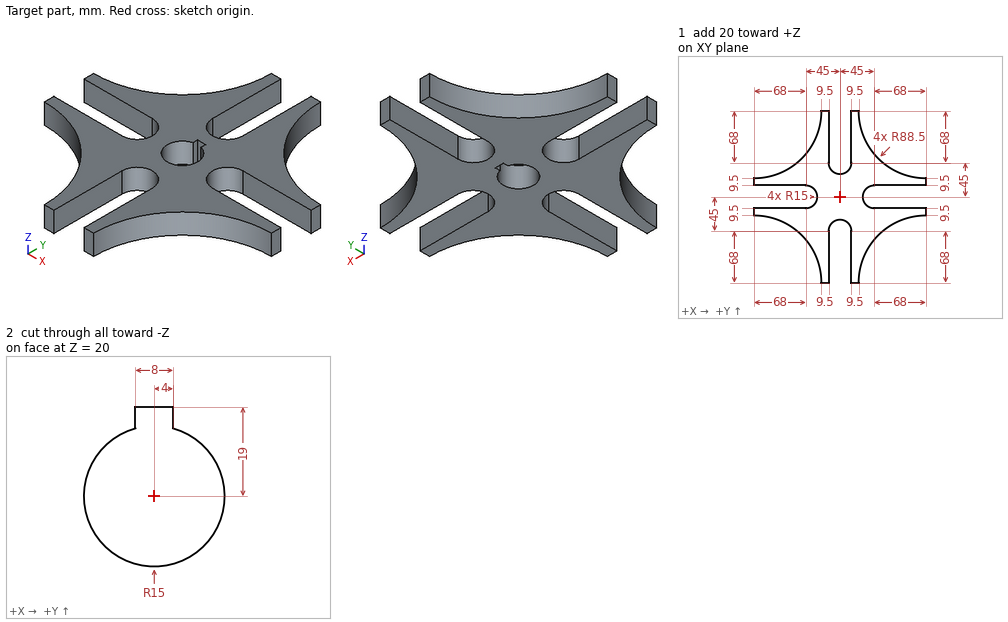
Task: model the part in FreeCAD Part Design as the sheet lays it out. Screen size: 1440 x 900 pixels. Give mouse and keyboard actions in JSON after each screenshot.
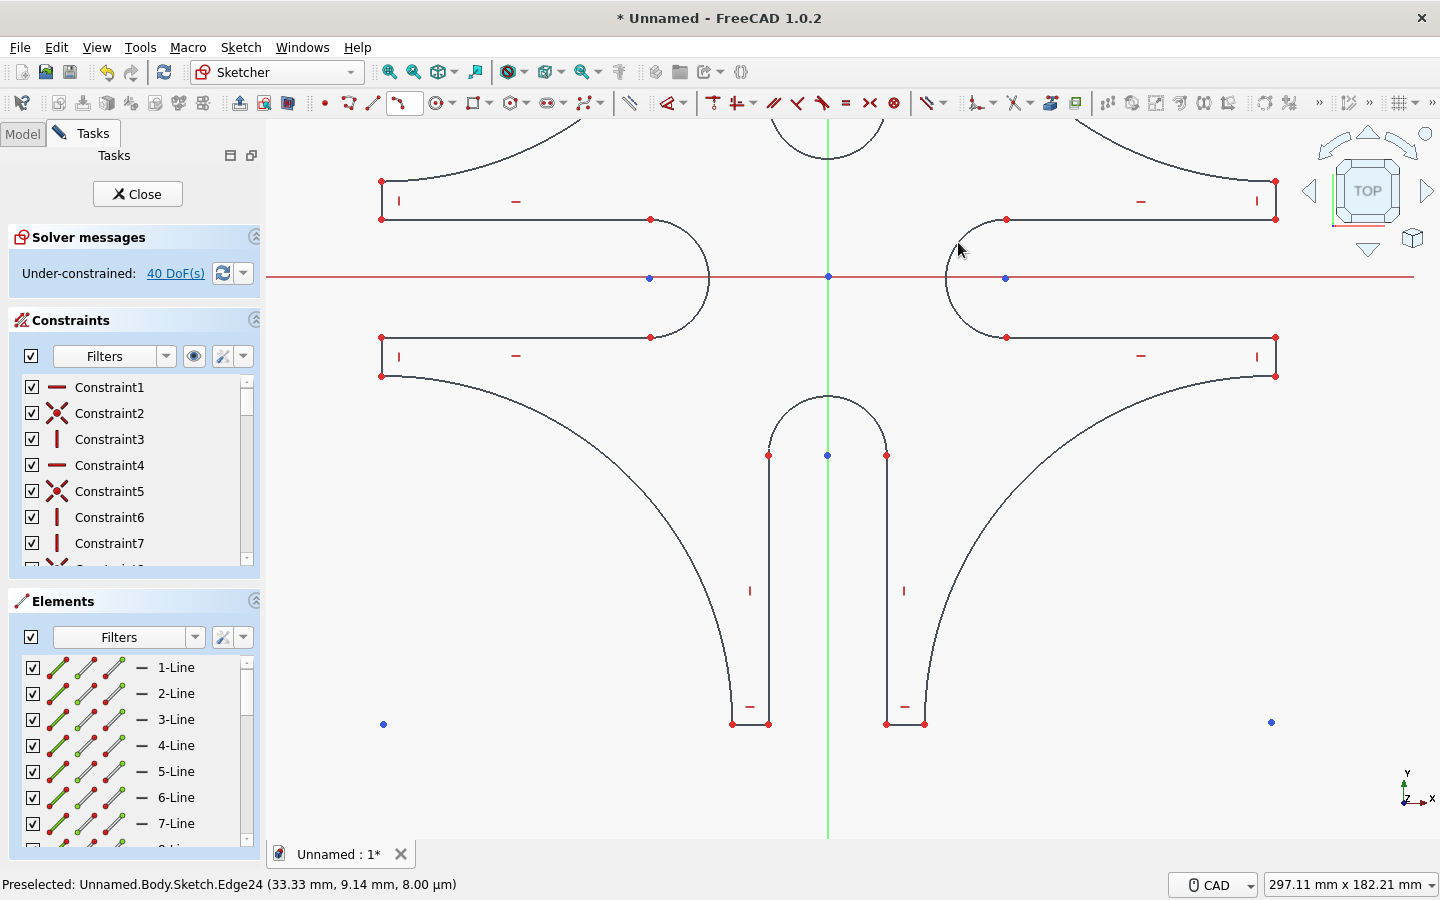
{"action": "left_click", "coordinate": [1087, 220]}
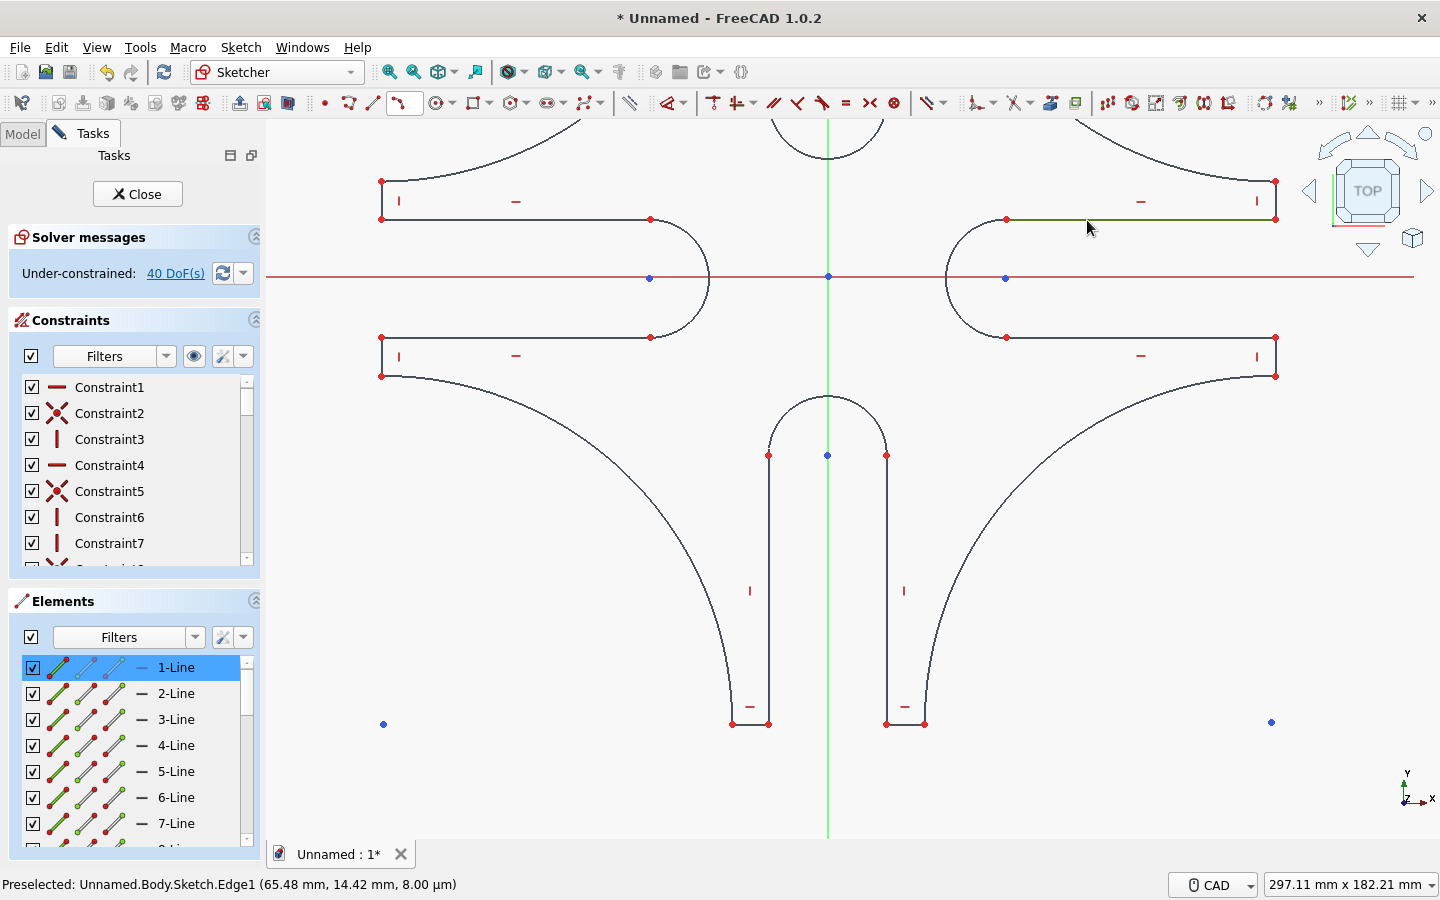
{"action": "left_click", "coordinate": [958, 244]}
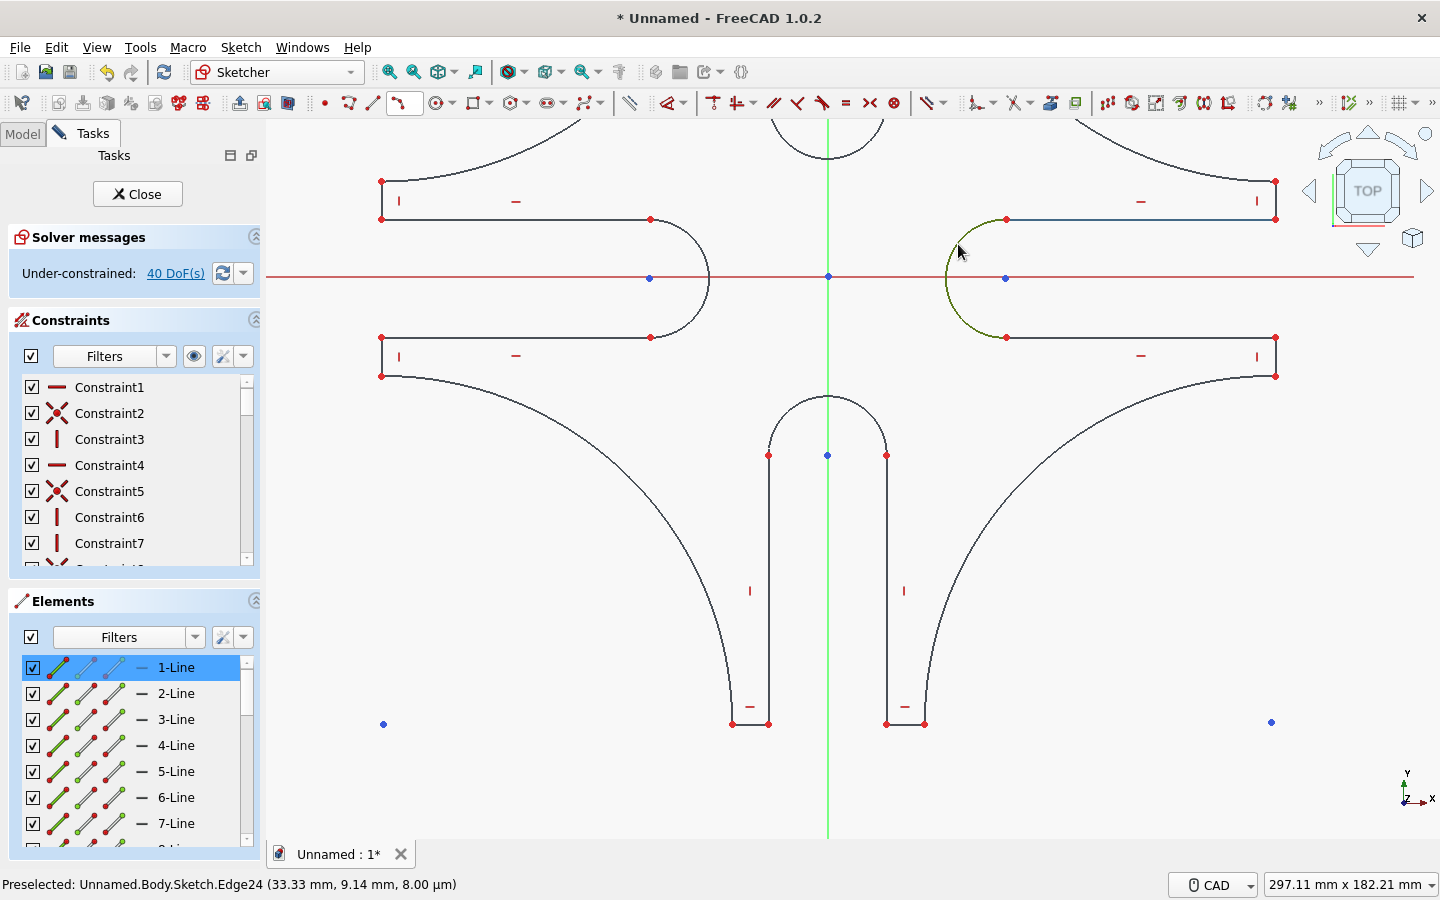
{"action": "left_click", "coordinate": [822, 104]}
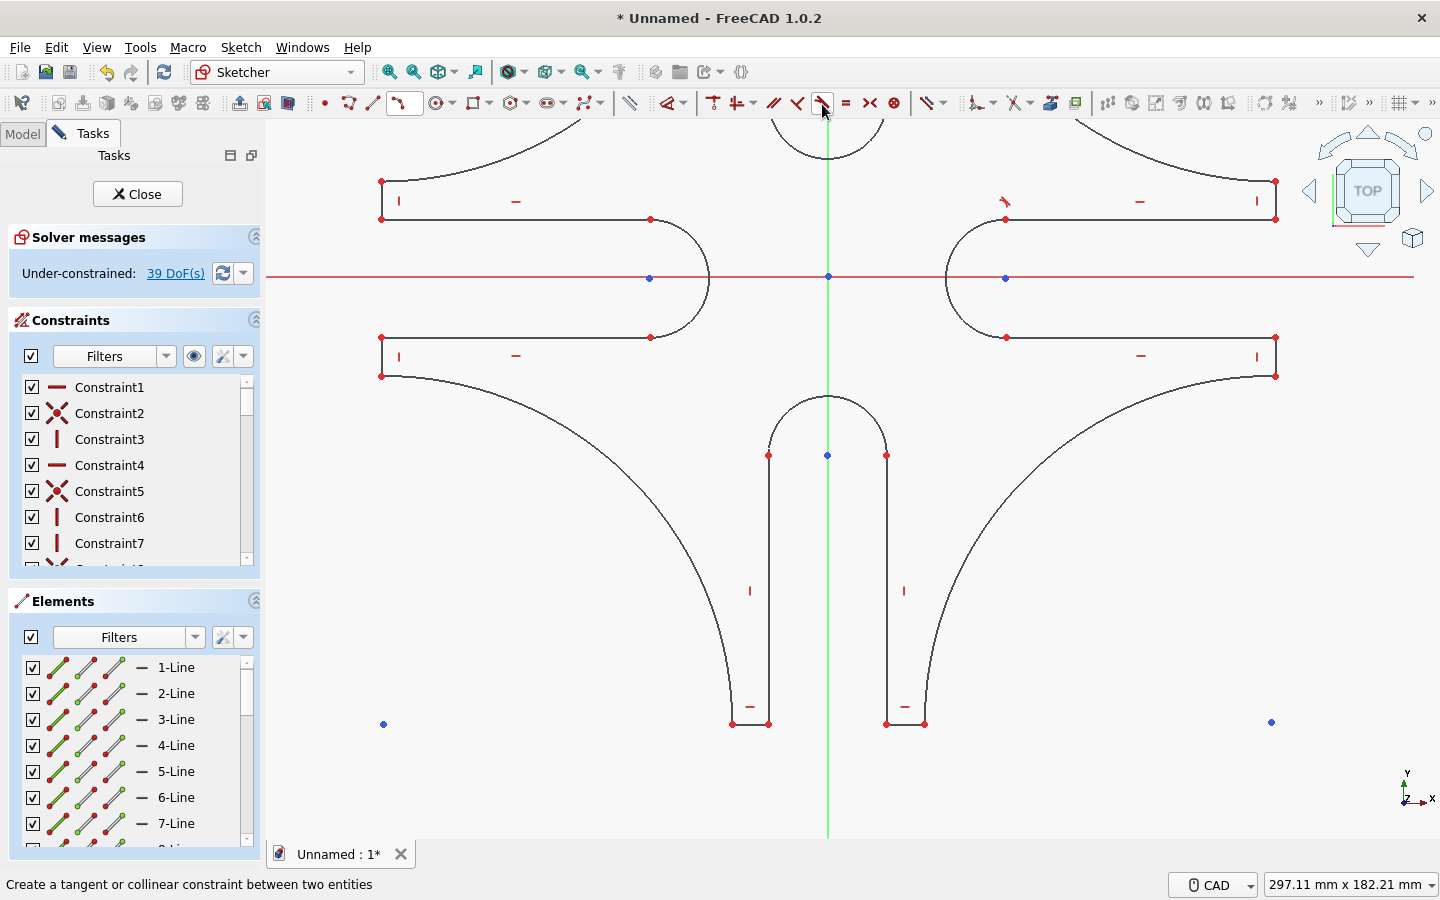
{"action": "scroll", "coordinate": [731, 725], "scroll_direction": "down", "scroll_amount": 3}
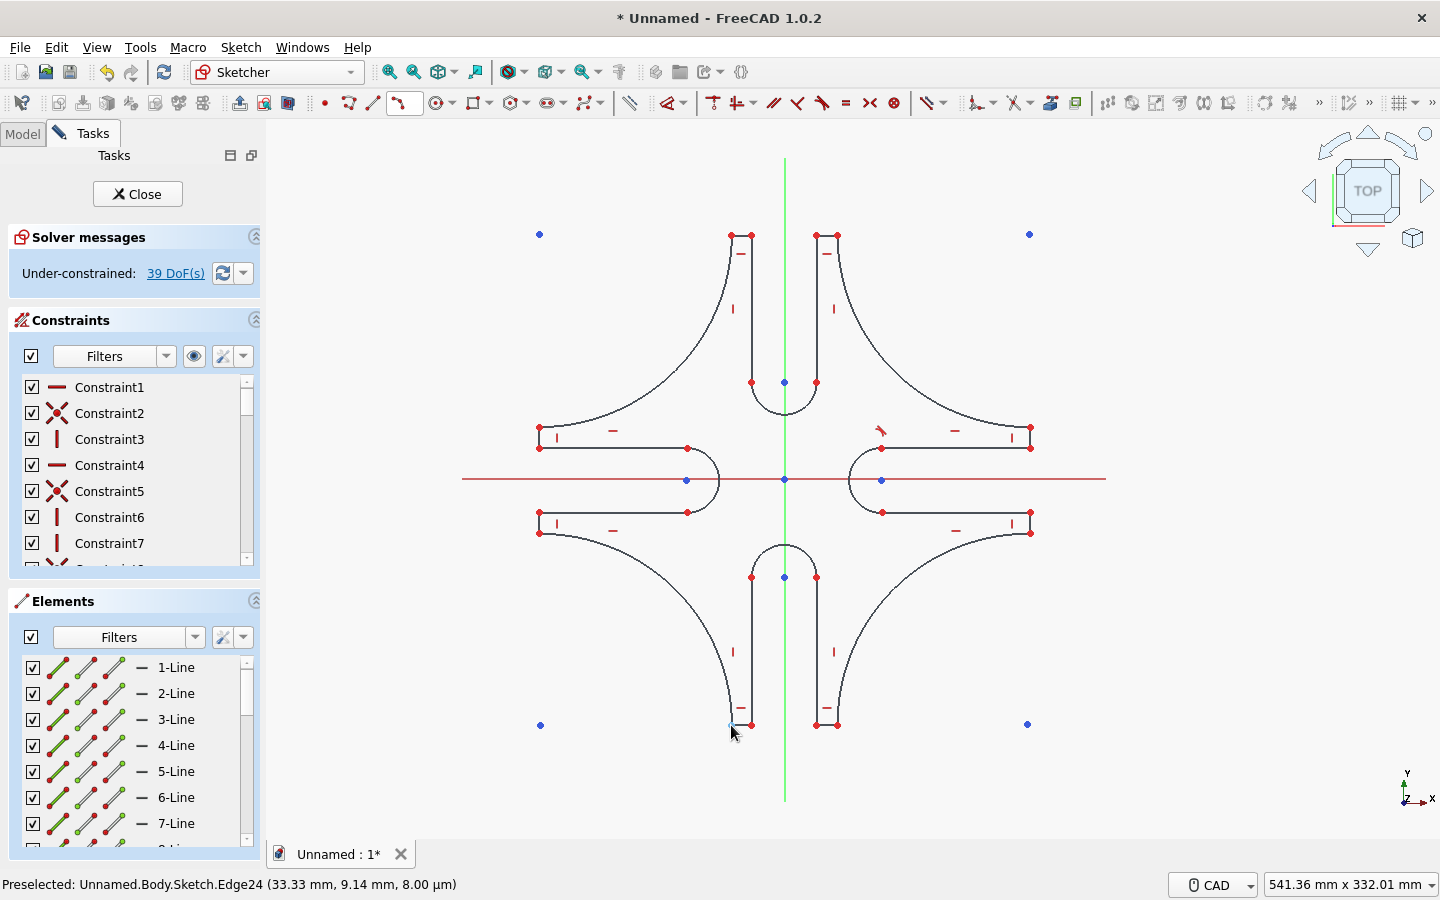
{"action": "left_click", "coordinate": [817, 280]}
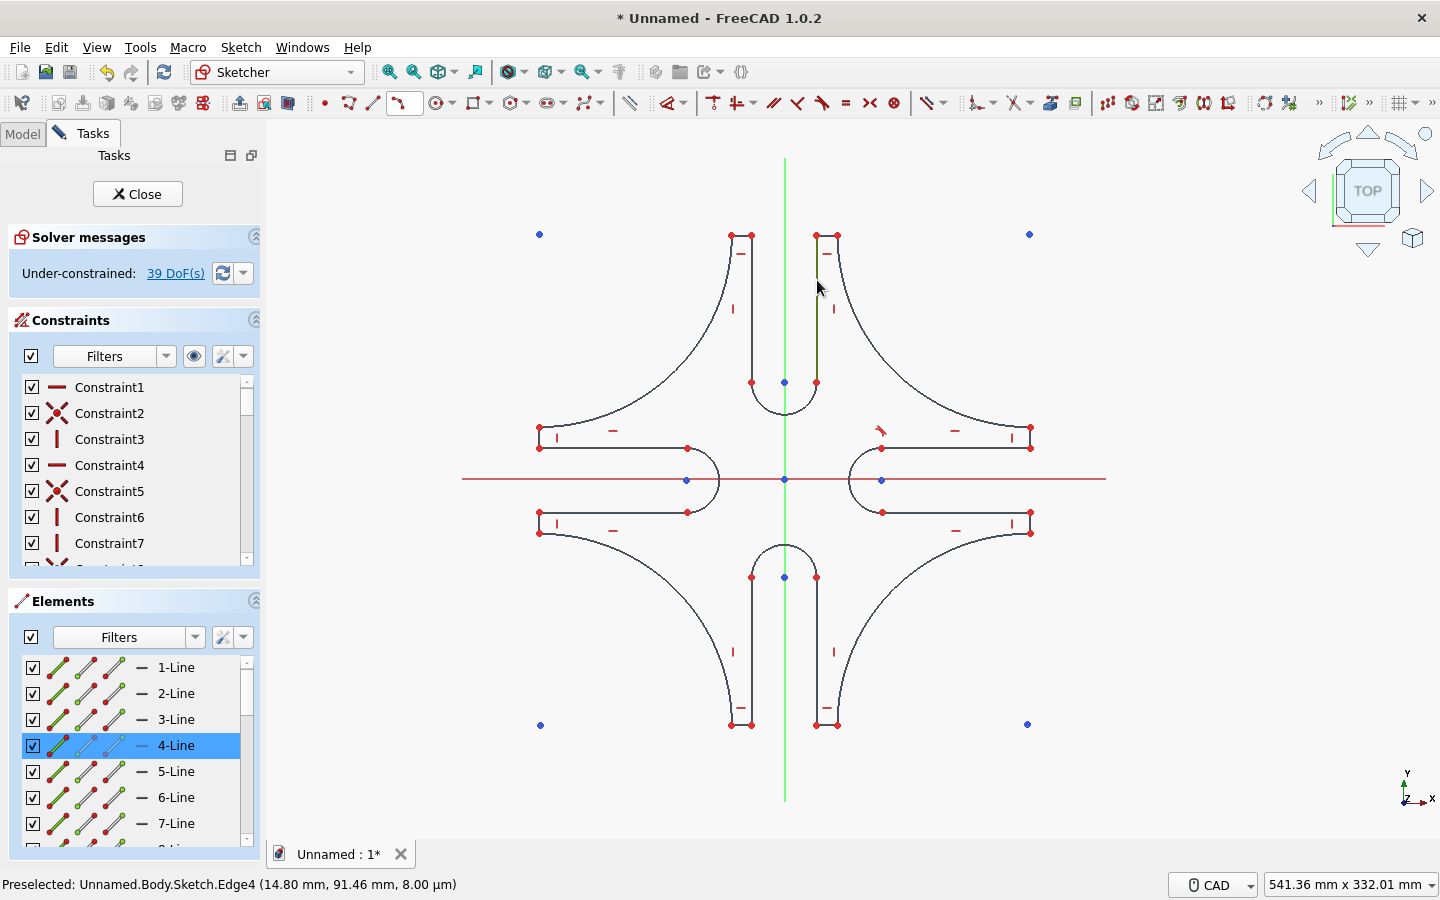
{"action": "left_click", "coordinate": [765, 408]}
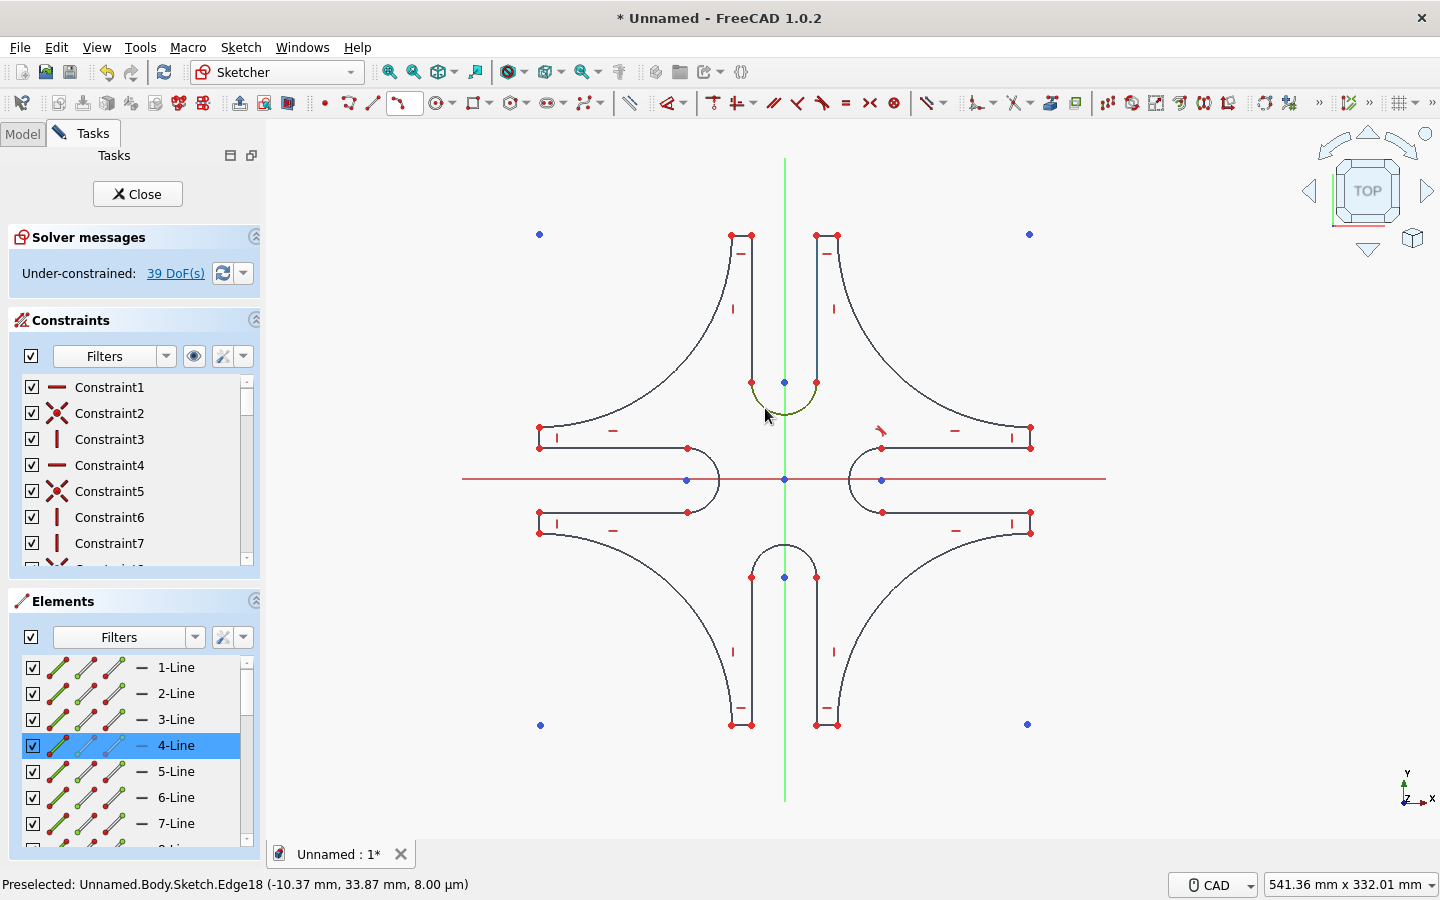
{"action": "left_click", "coordinate": [822, 104]}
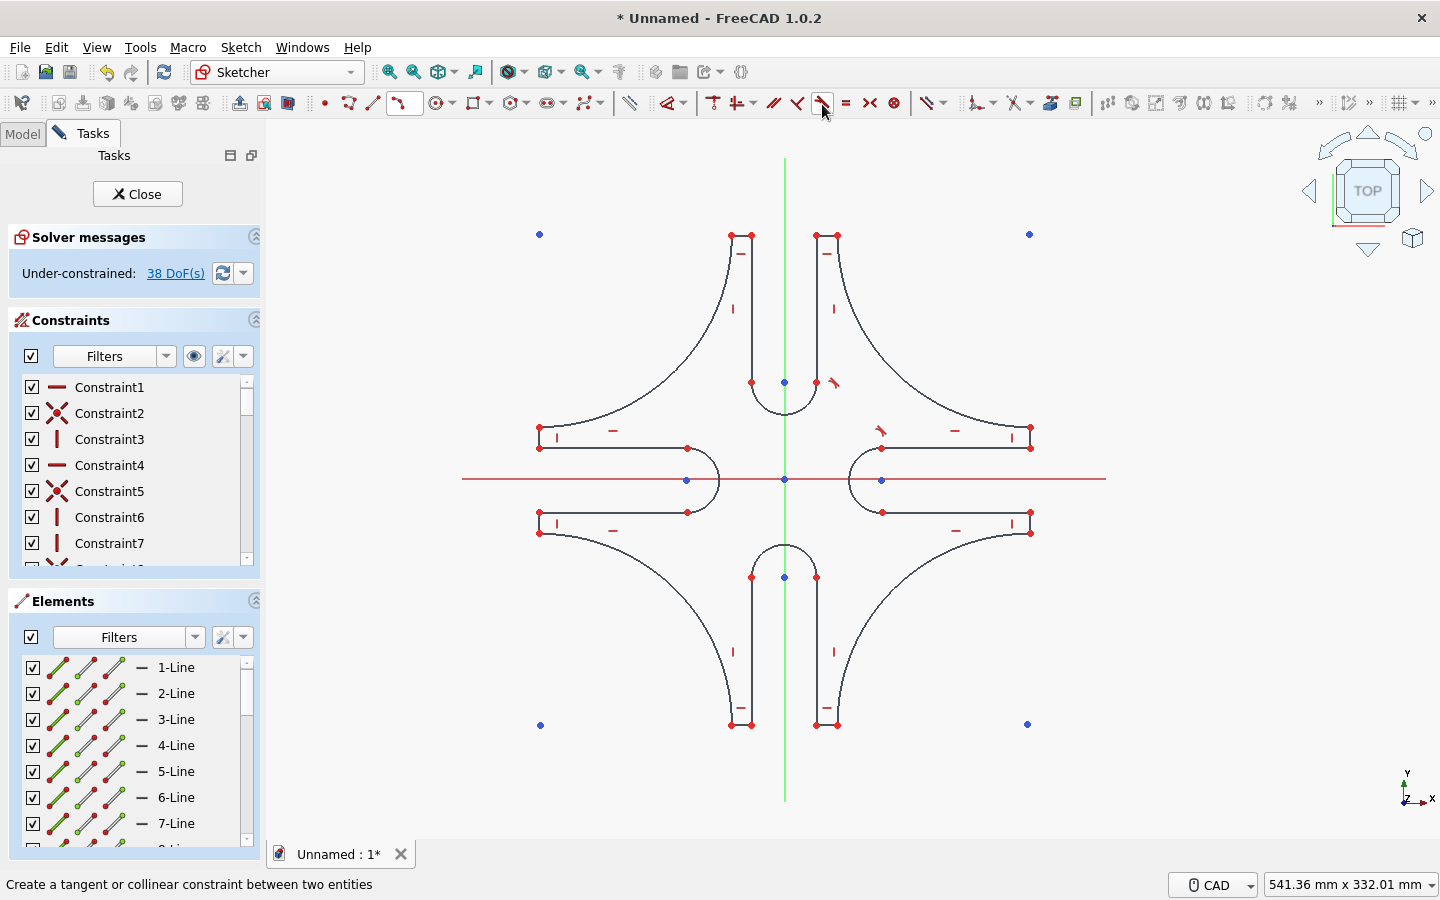
{"action": "left_click", "coordinate": [752, 338]}